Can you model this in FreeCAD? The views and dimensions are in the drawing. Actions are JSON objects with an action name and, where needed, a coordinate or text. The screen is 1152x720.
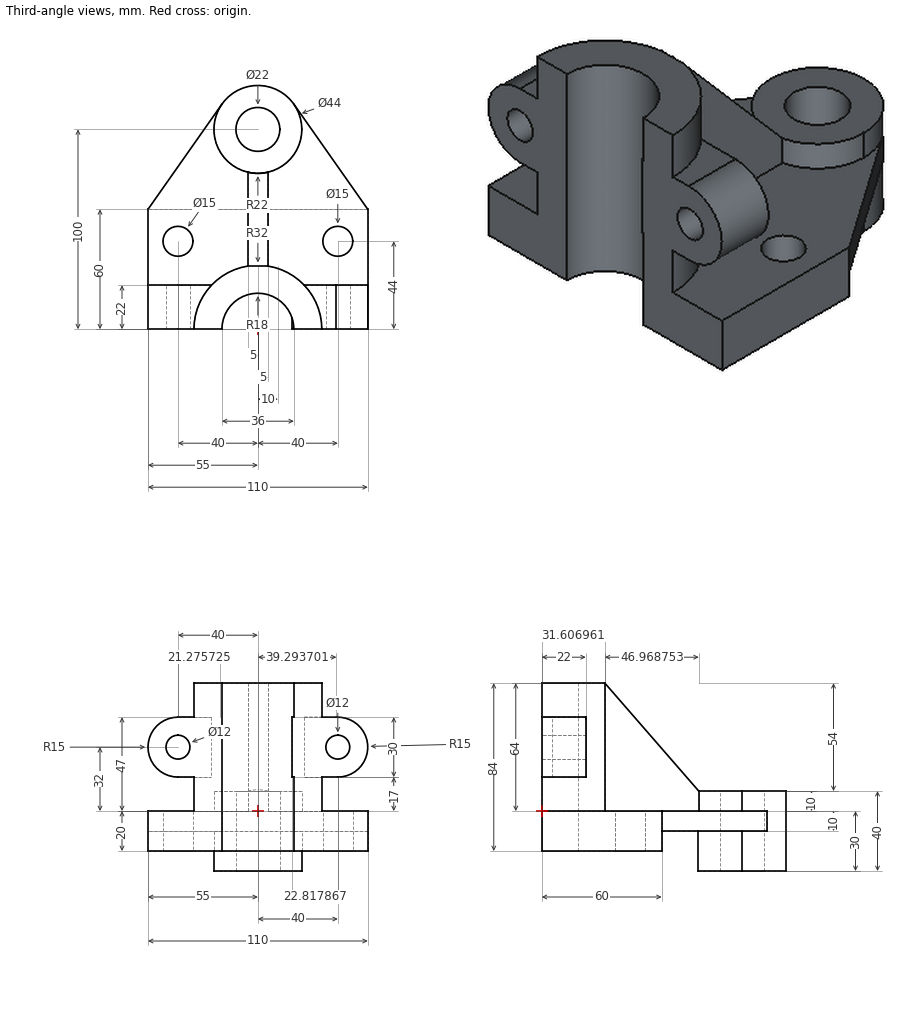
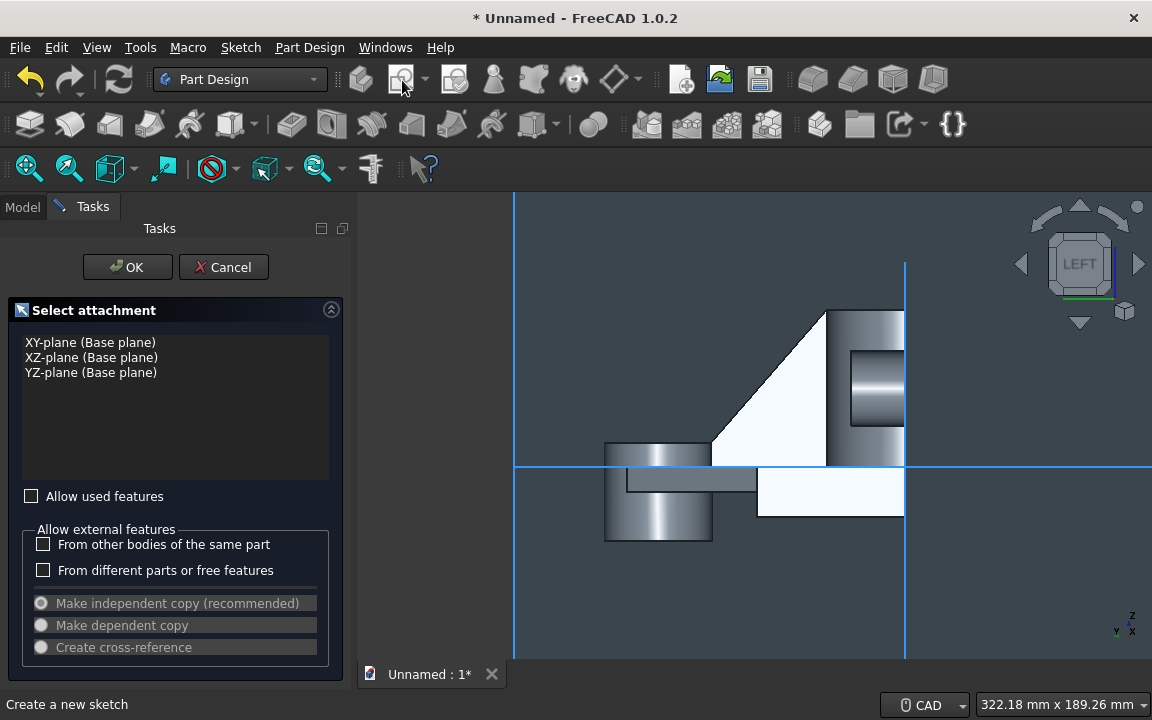
{"action": "left_click", "coordinate": [82, 342]}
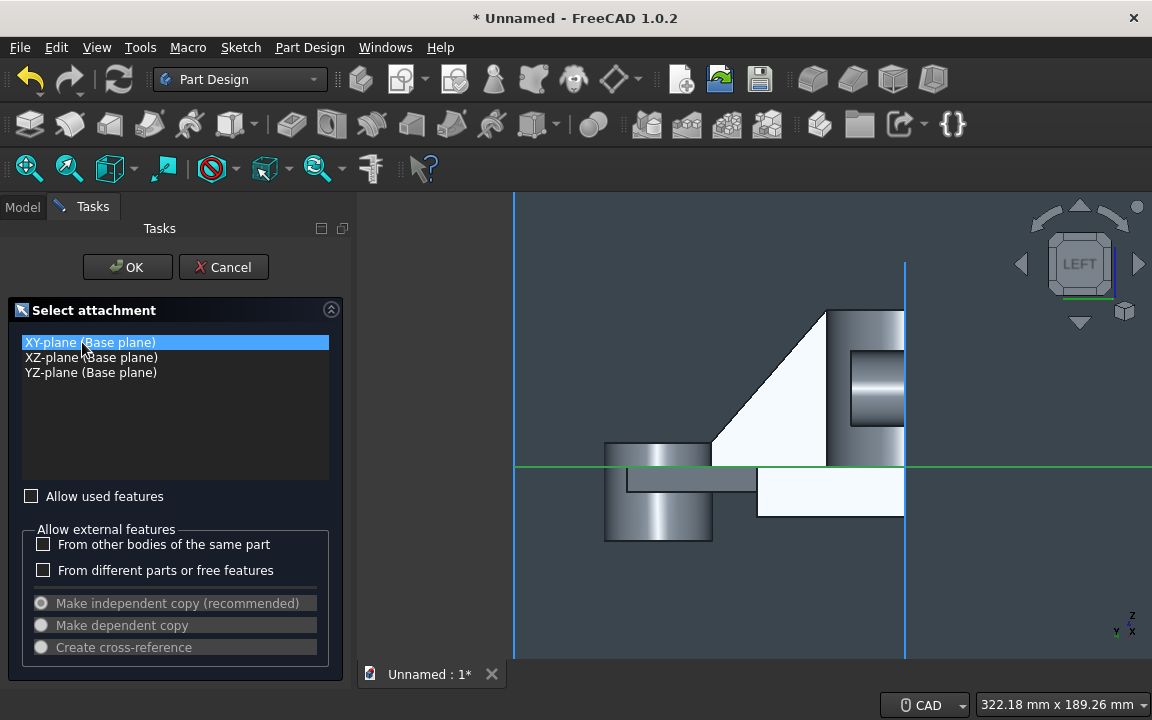
{"action": "left_click", "coordinate": [128, 267]}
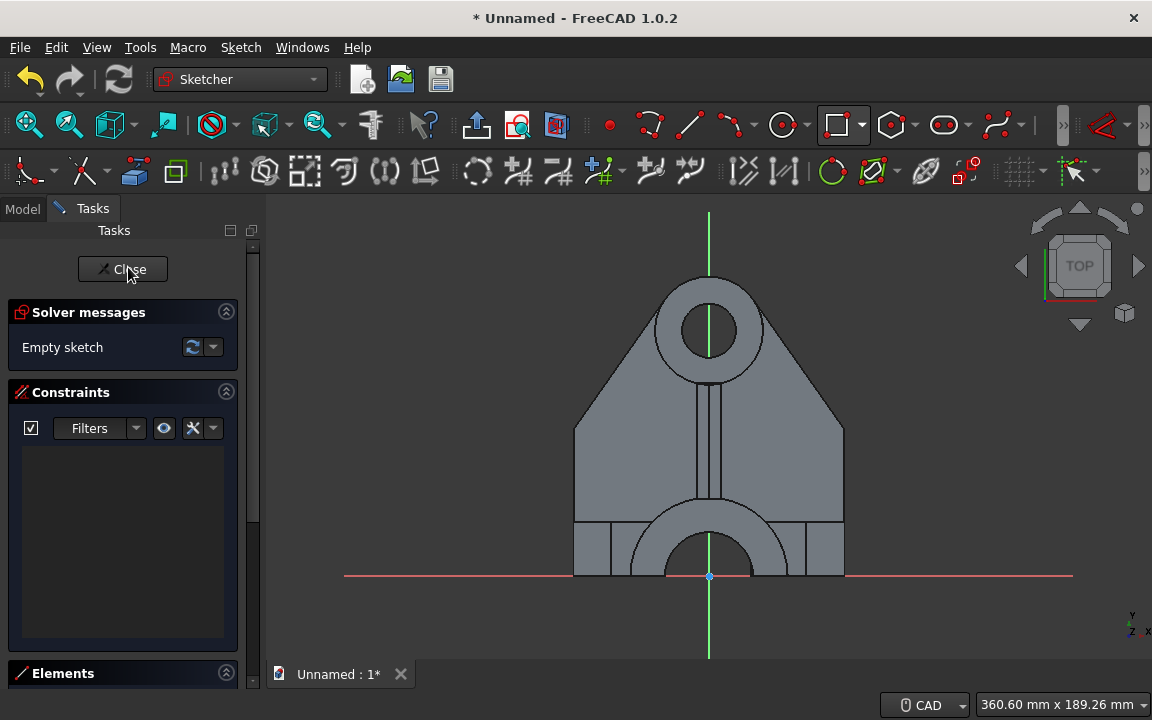
{"action": "left_click", "coordinate": [558, 126]}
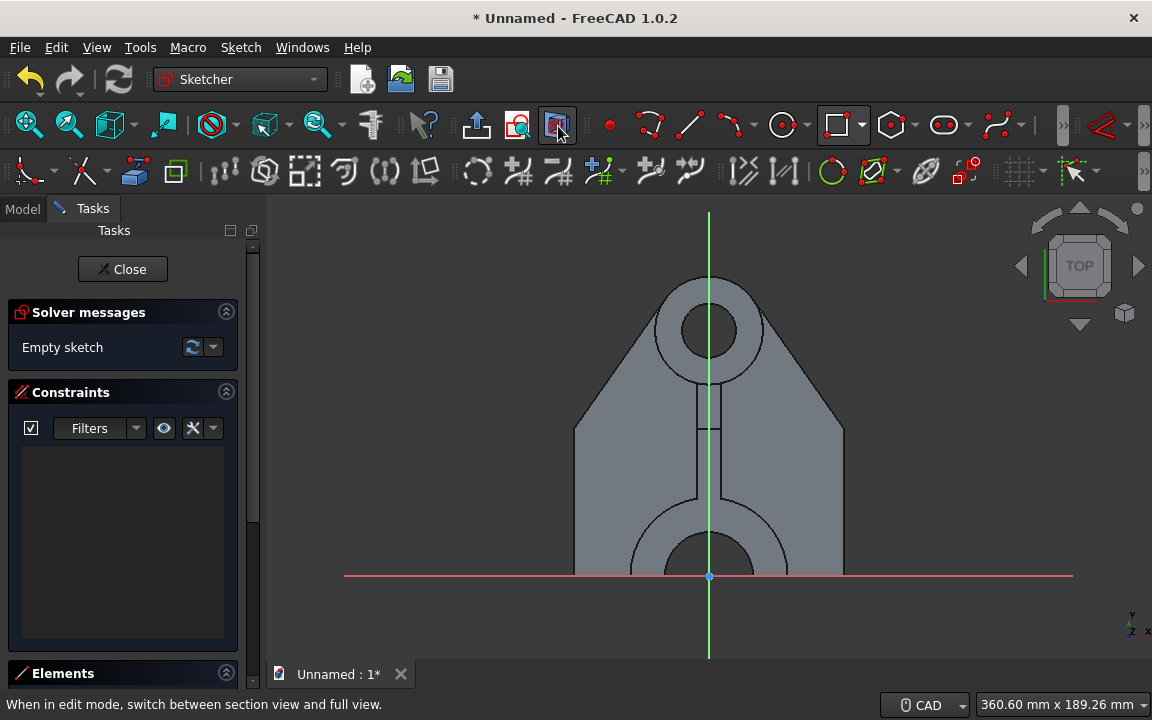
{"action": "scroll", "coordinate": [833, 475], "scroll_direction": "up", "scroll_amount": 10}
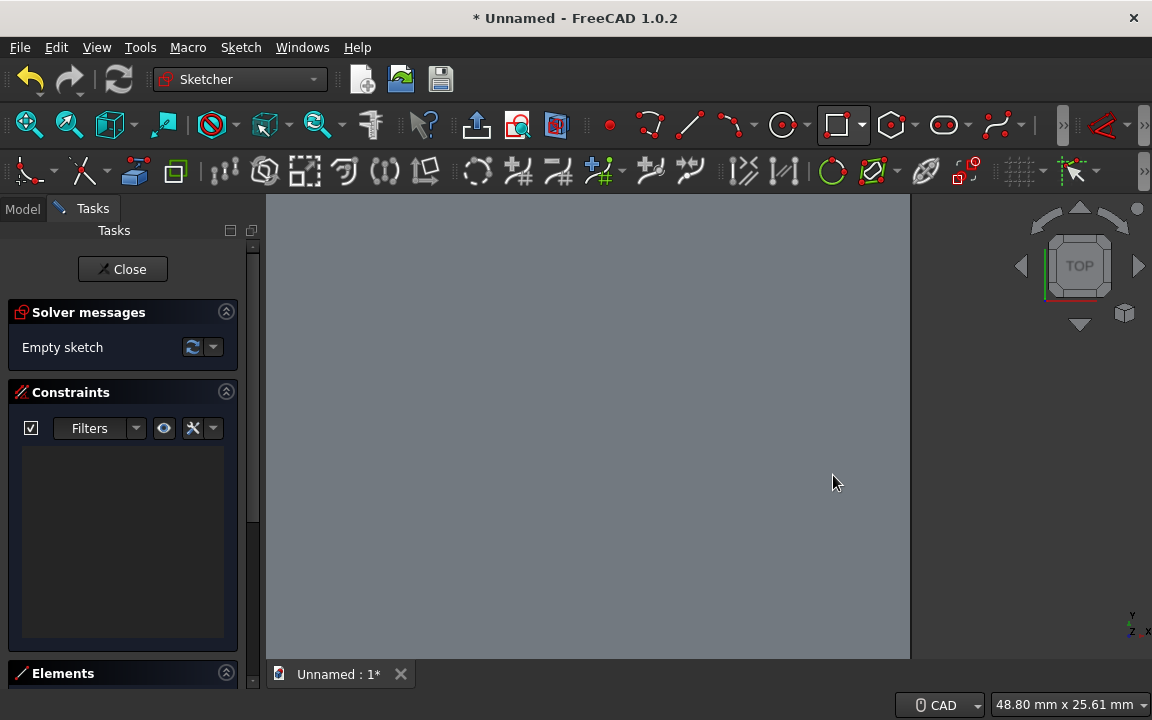
{"action": "left_click", "coordinate": [784, 126]}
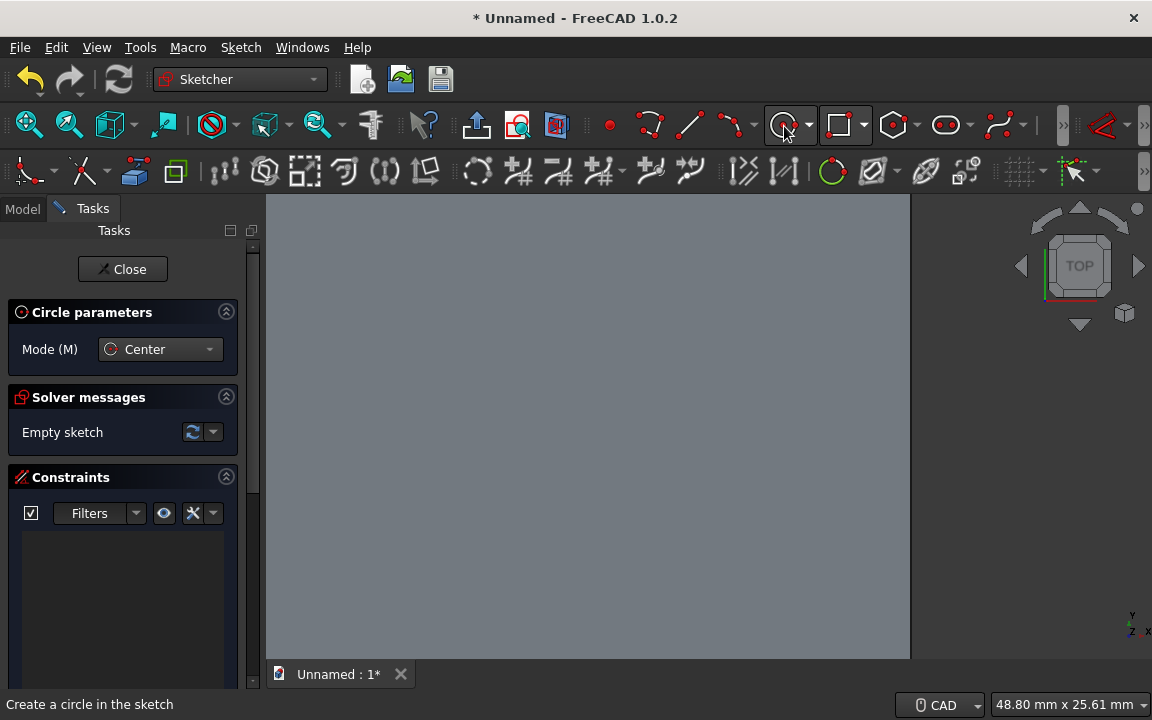
{"action": "left_click", "coordinate": [639, 421]}
{"action": "left_click", "coordinate": [735, 325]}
{"action": "key", "text": "Escape"}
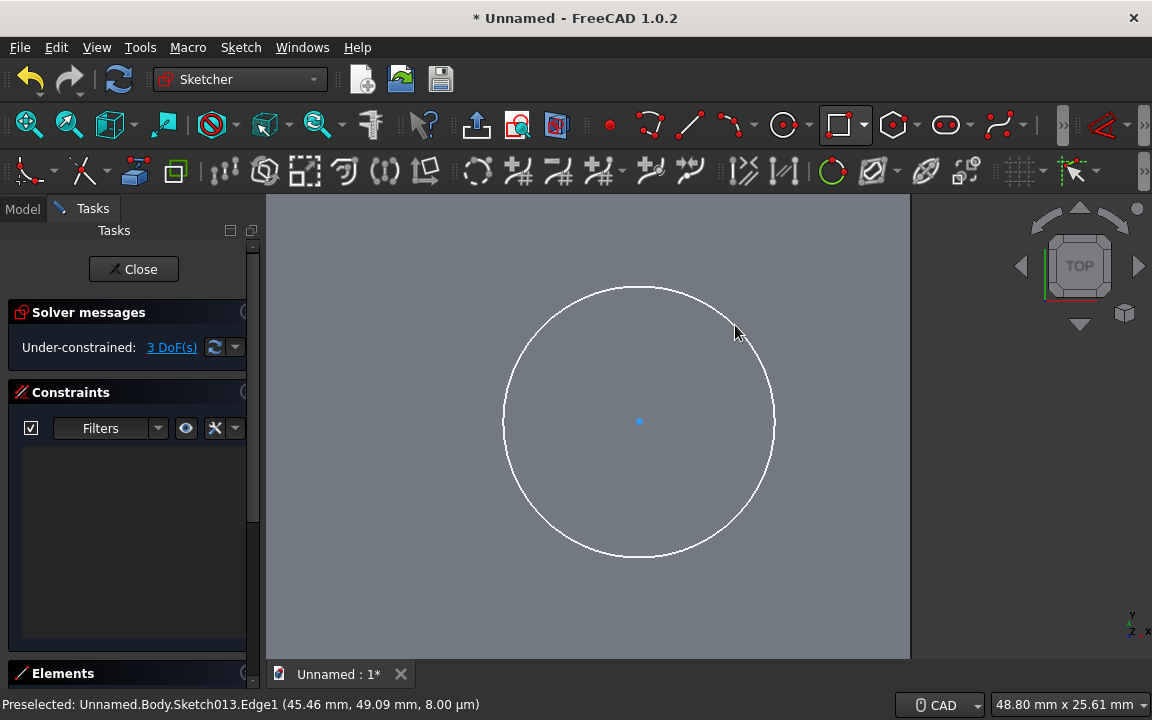
{"action": "left_click", "coordinate": [1102, 126]}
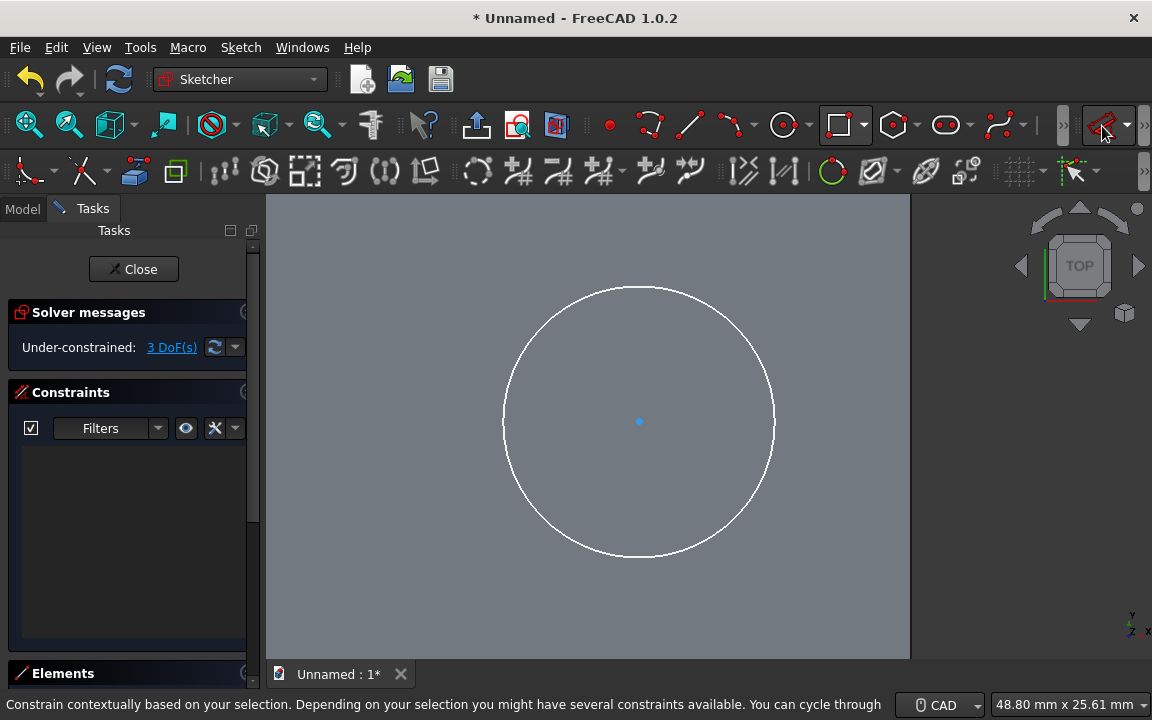
{"action": "left_click", "coordinate": [735, 326]}
{"action": "left_click", "coordinate": [758, 303]}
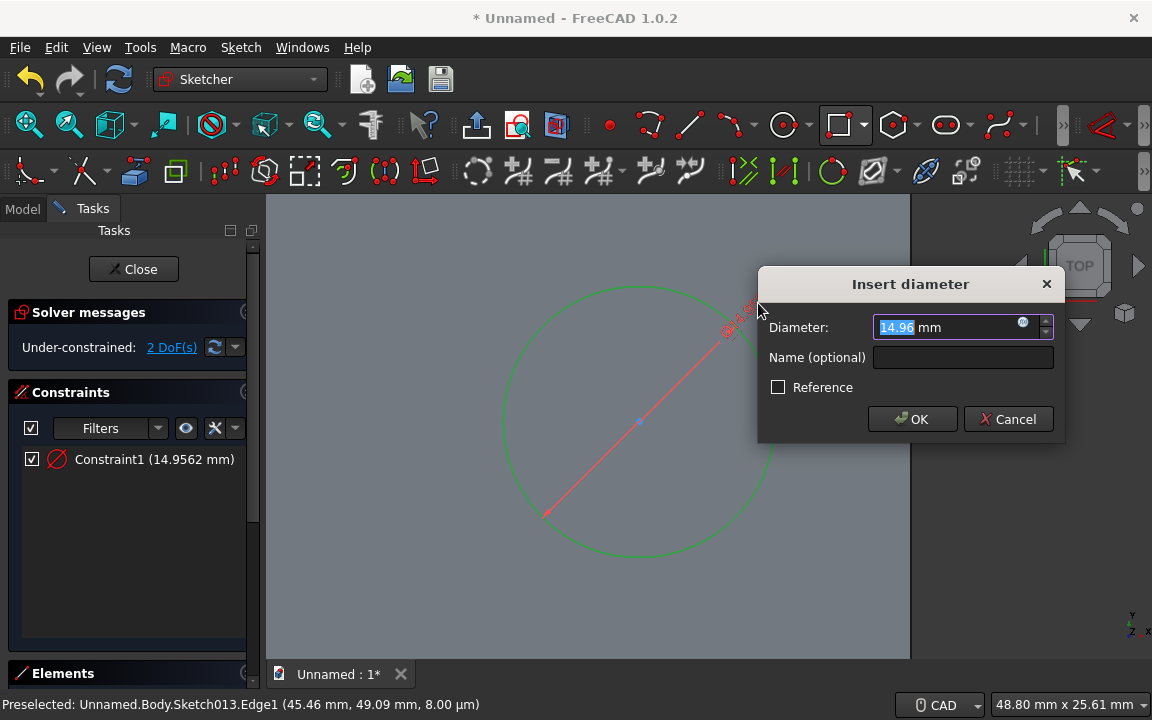
{"action": "type", "text": "15"}
{"action": "key", "text": "Return"}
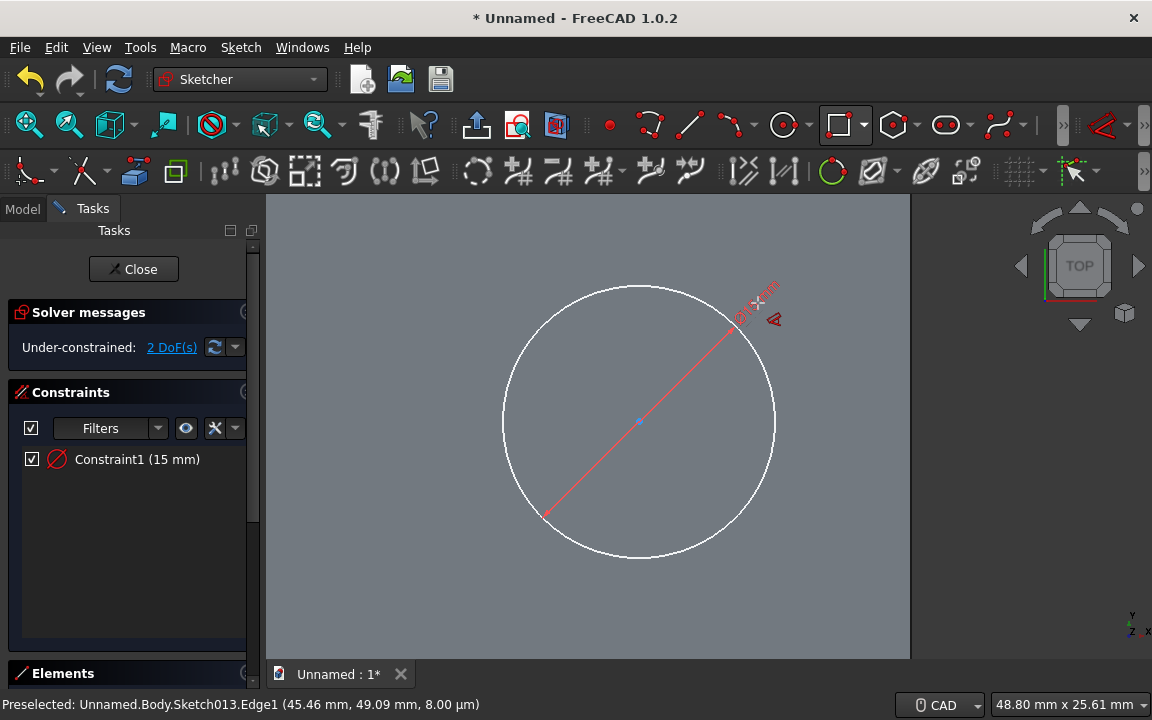
{"action": "left_click", "coordinate": [639, 422]}
{"action": "left_click", "coordinate": [467, 388]}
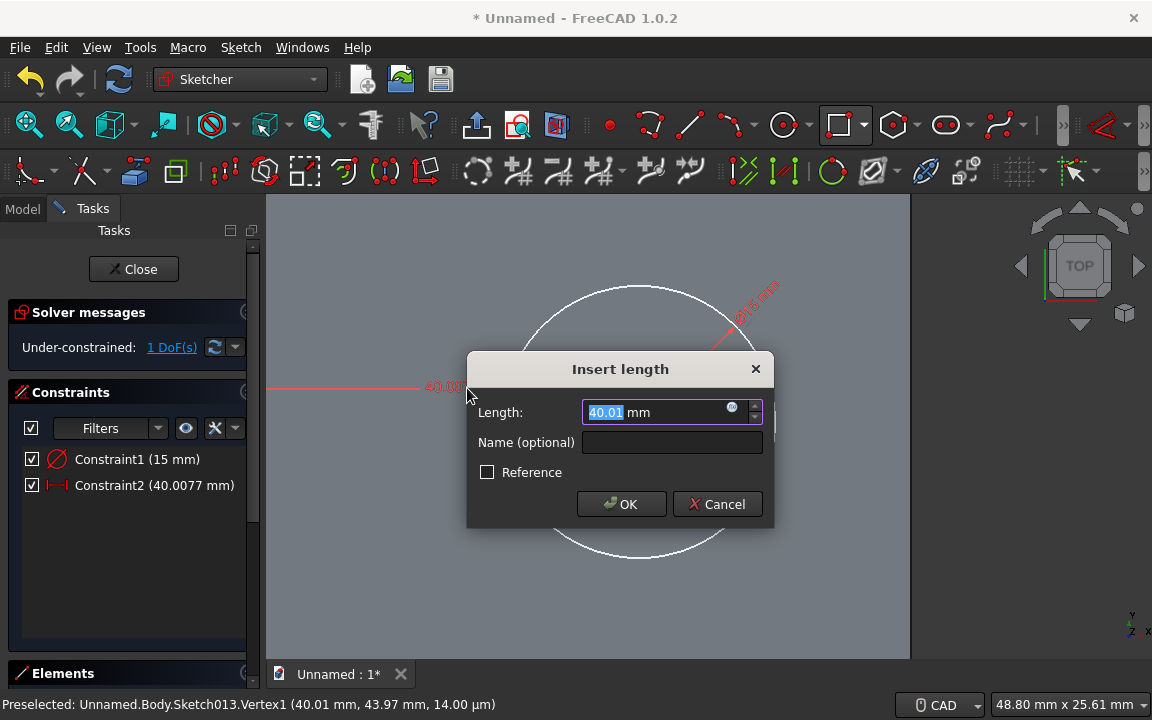
{"action": "type", "text": "40"}
{"action": "key", "text": "Return"}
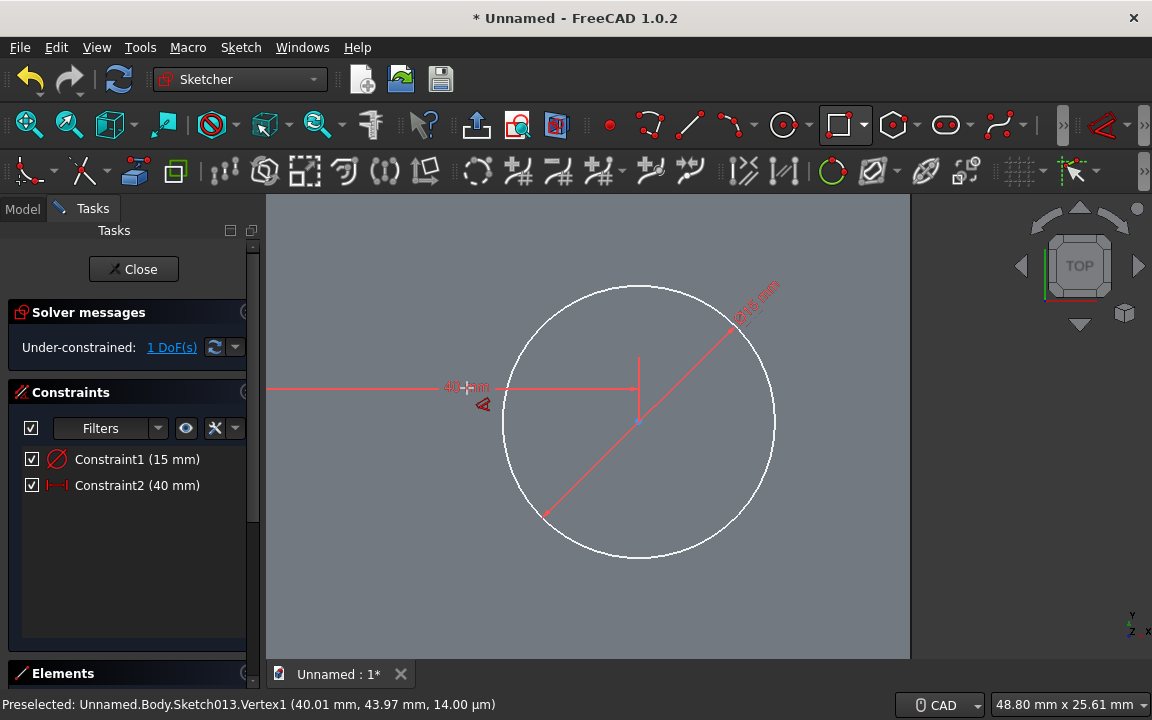
{"action": "left_click", "coordinate": [639, 422]}
{"action": "left_click", "coordinate": [673, 526]}